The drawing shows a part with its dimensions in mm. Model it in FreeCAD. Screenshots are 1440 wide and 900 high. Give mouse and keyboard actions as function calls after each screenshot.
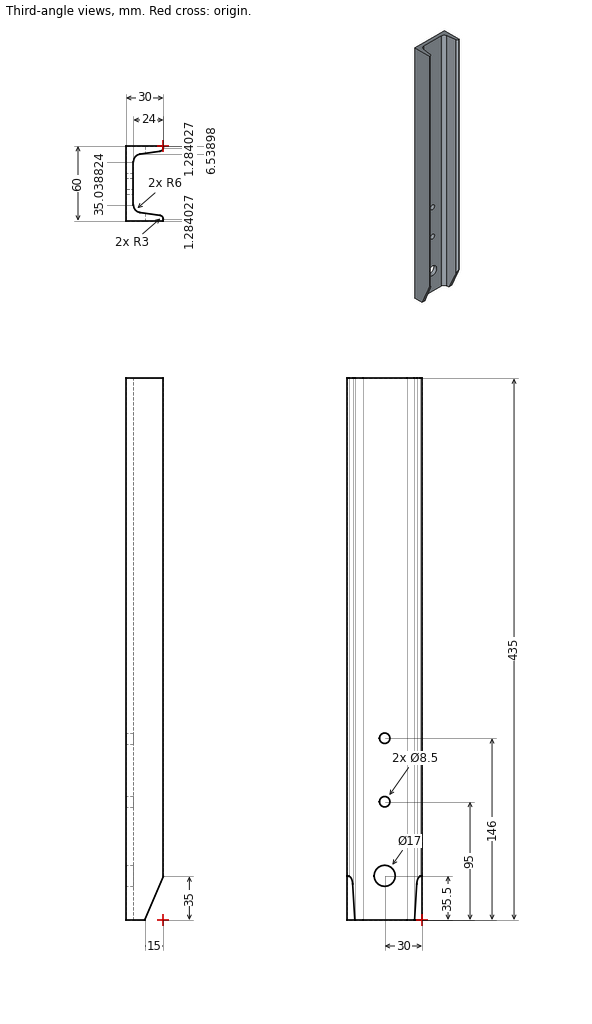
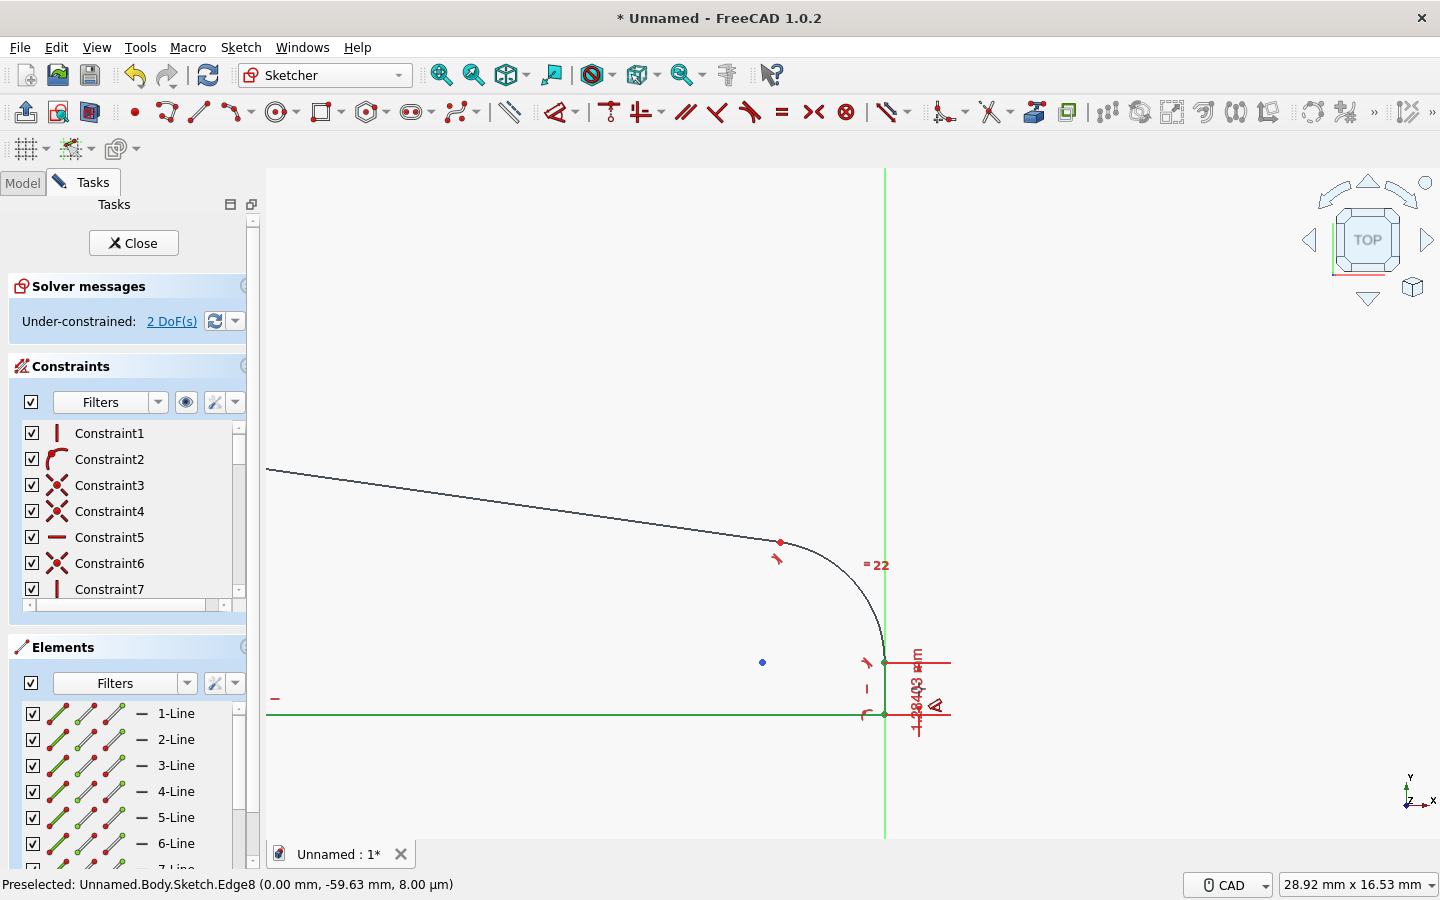
scroll(885, 703, down, 9)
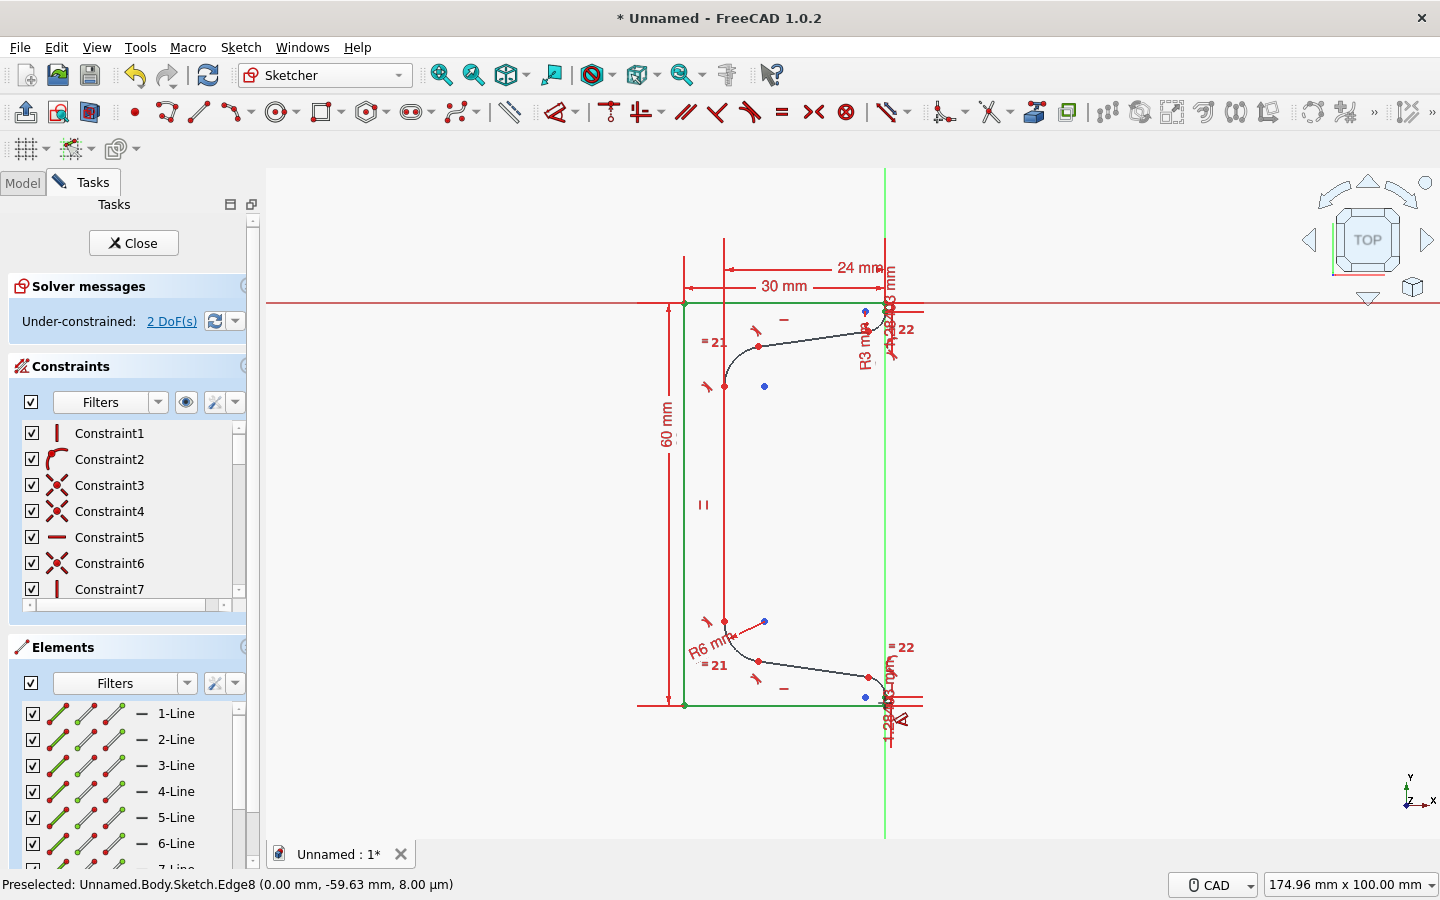
click(759, 347)
click(725, 325)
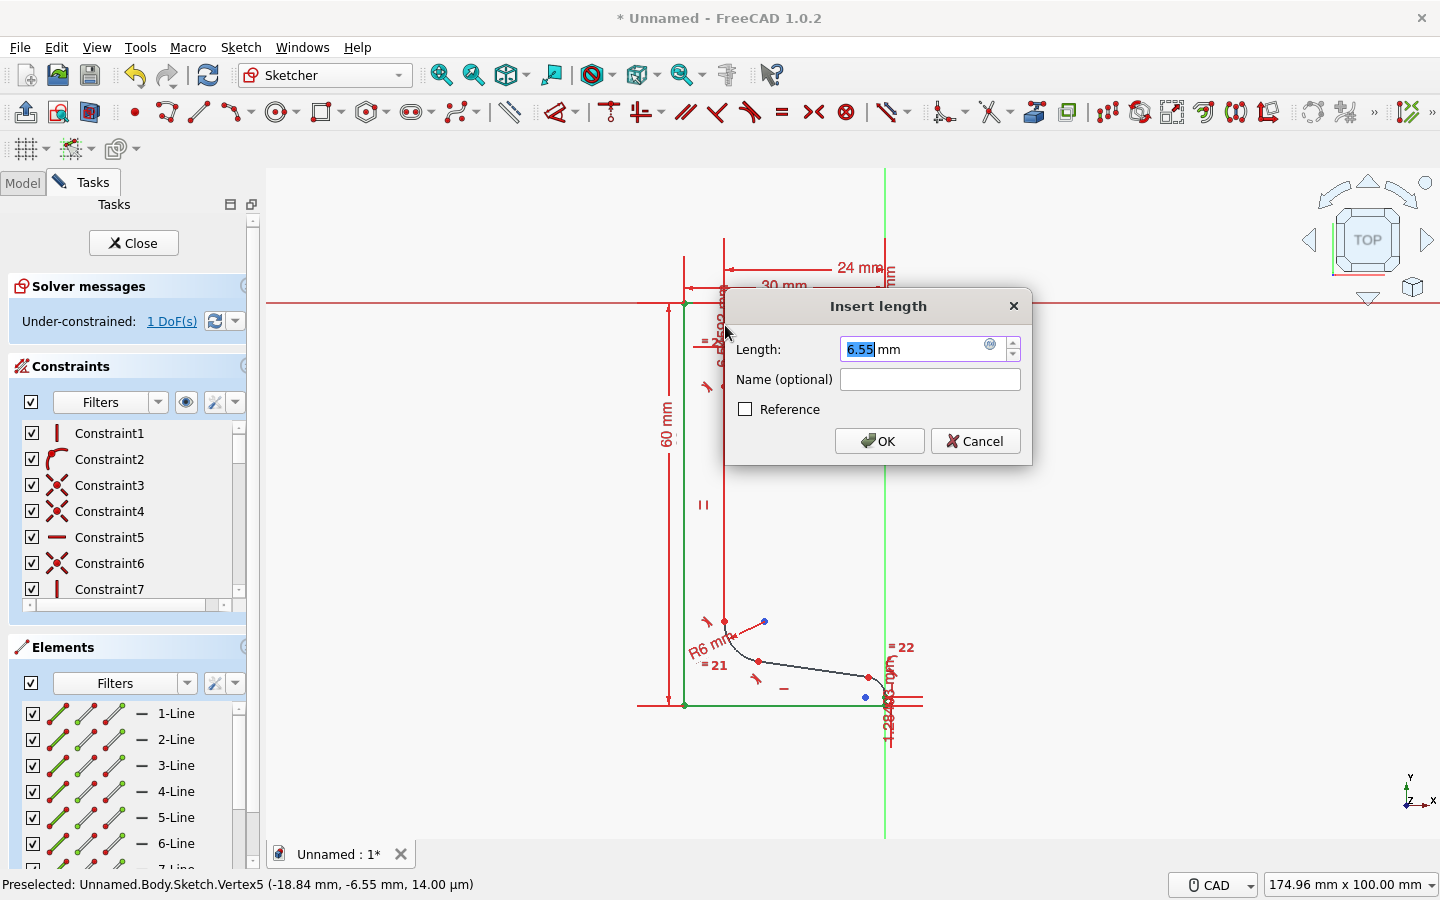
text(6.53898)
key(Return)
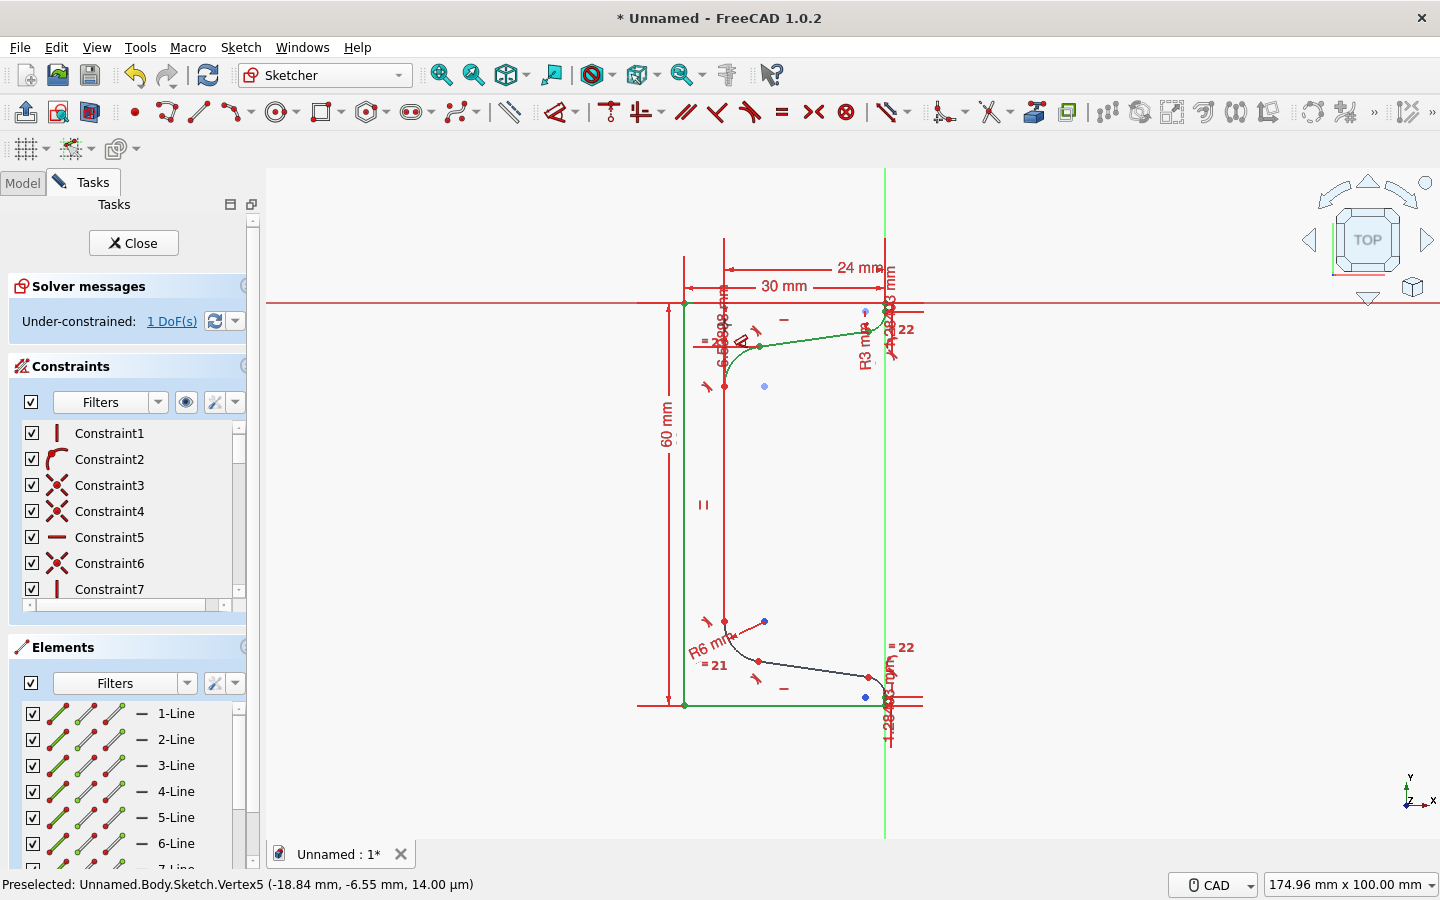
click(724, 551)
click(758, 504)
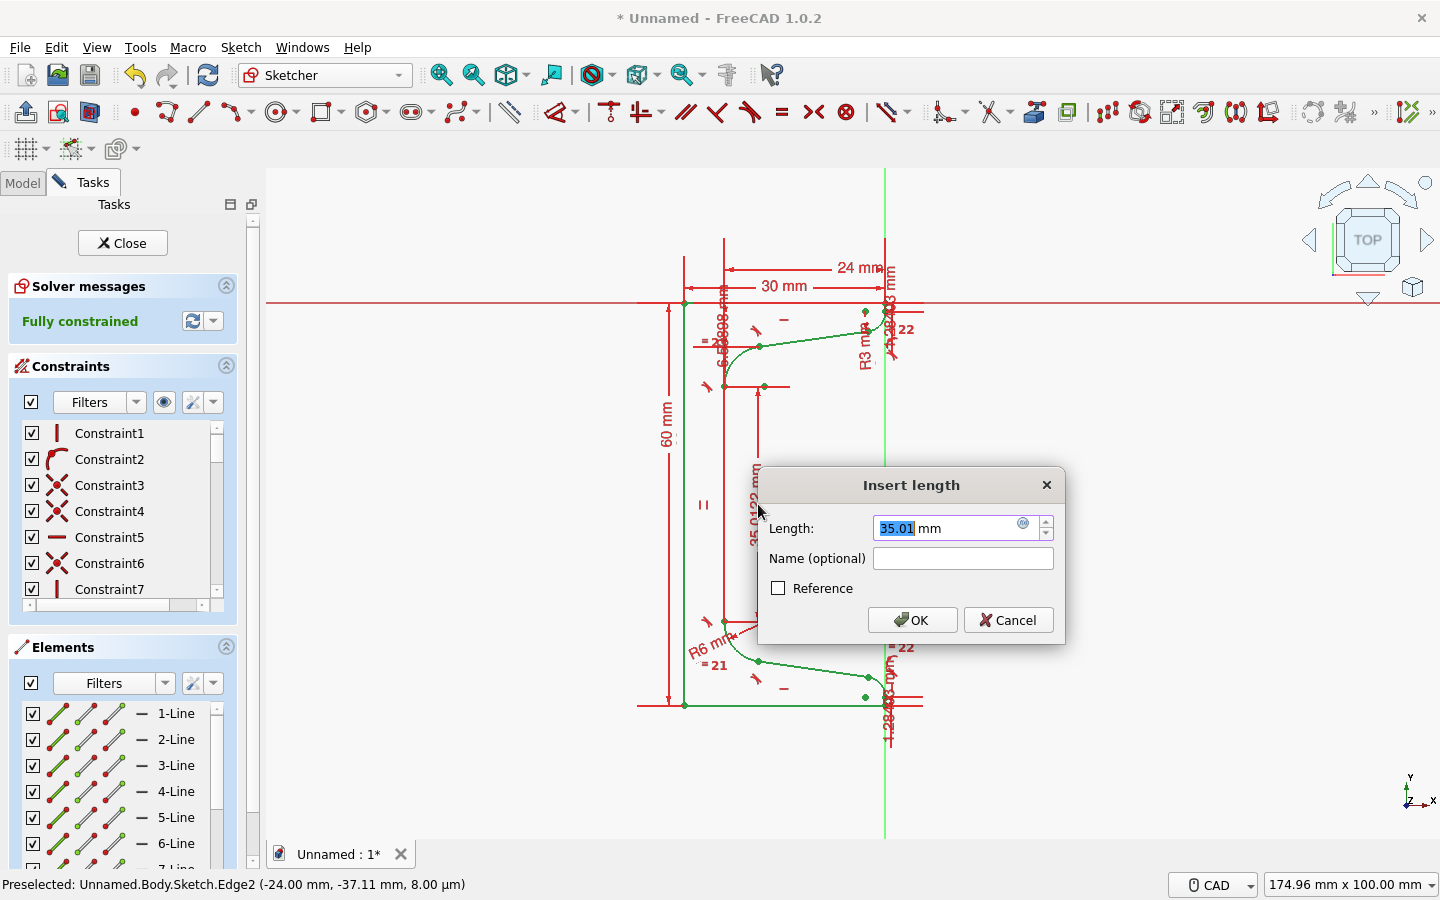
text(35.038824)
key(Return)
key(Escape)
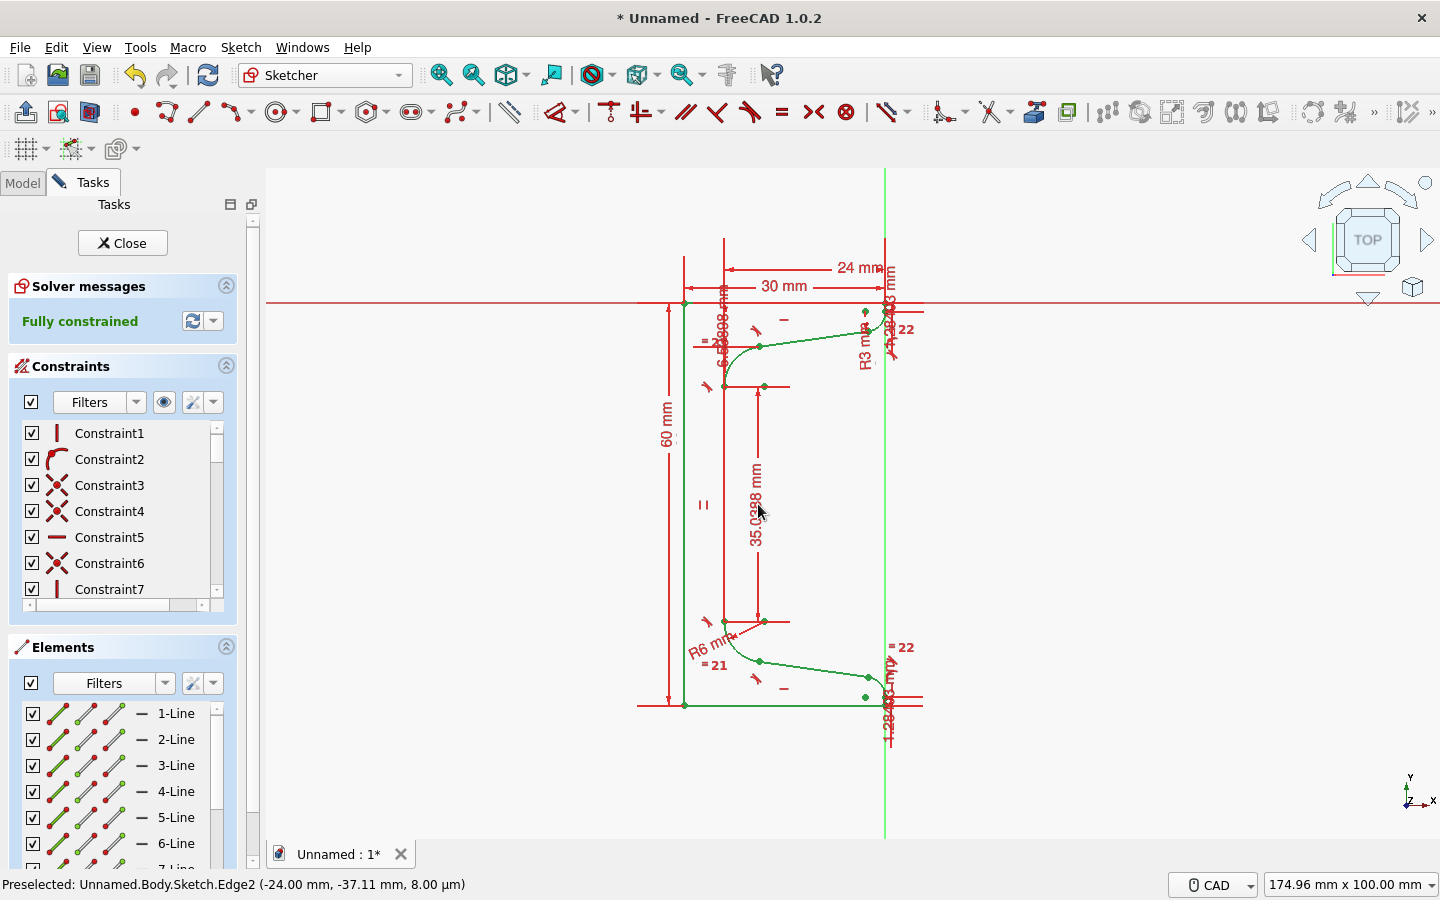
click(123, 243)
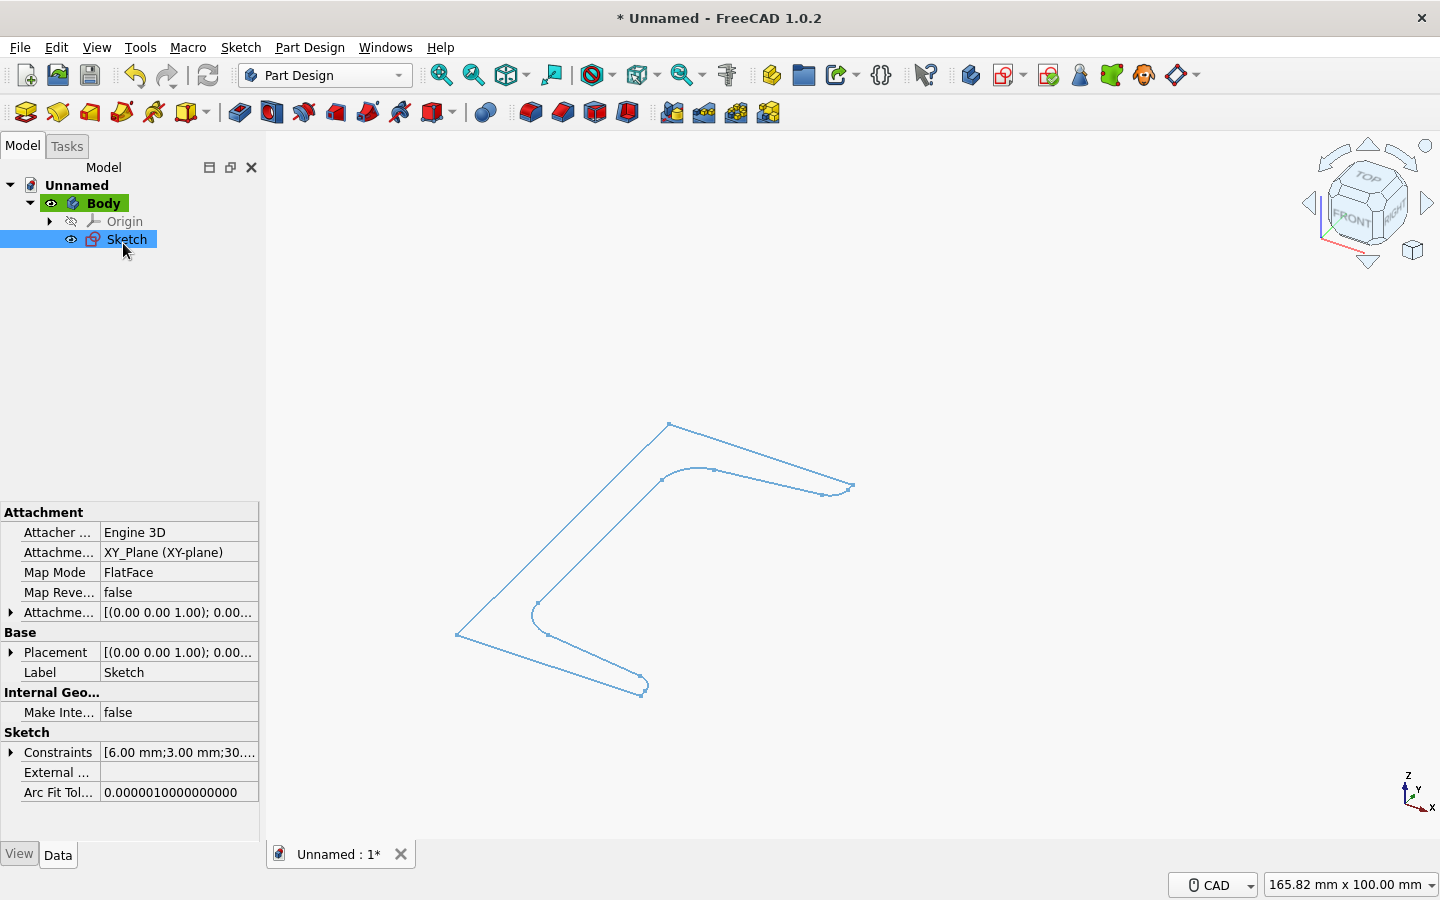
click(26, 112)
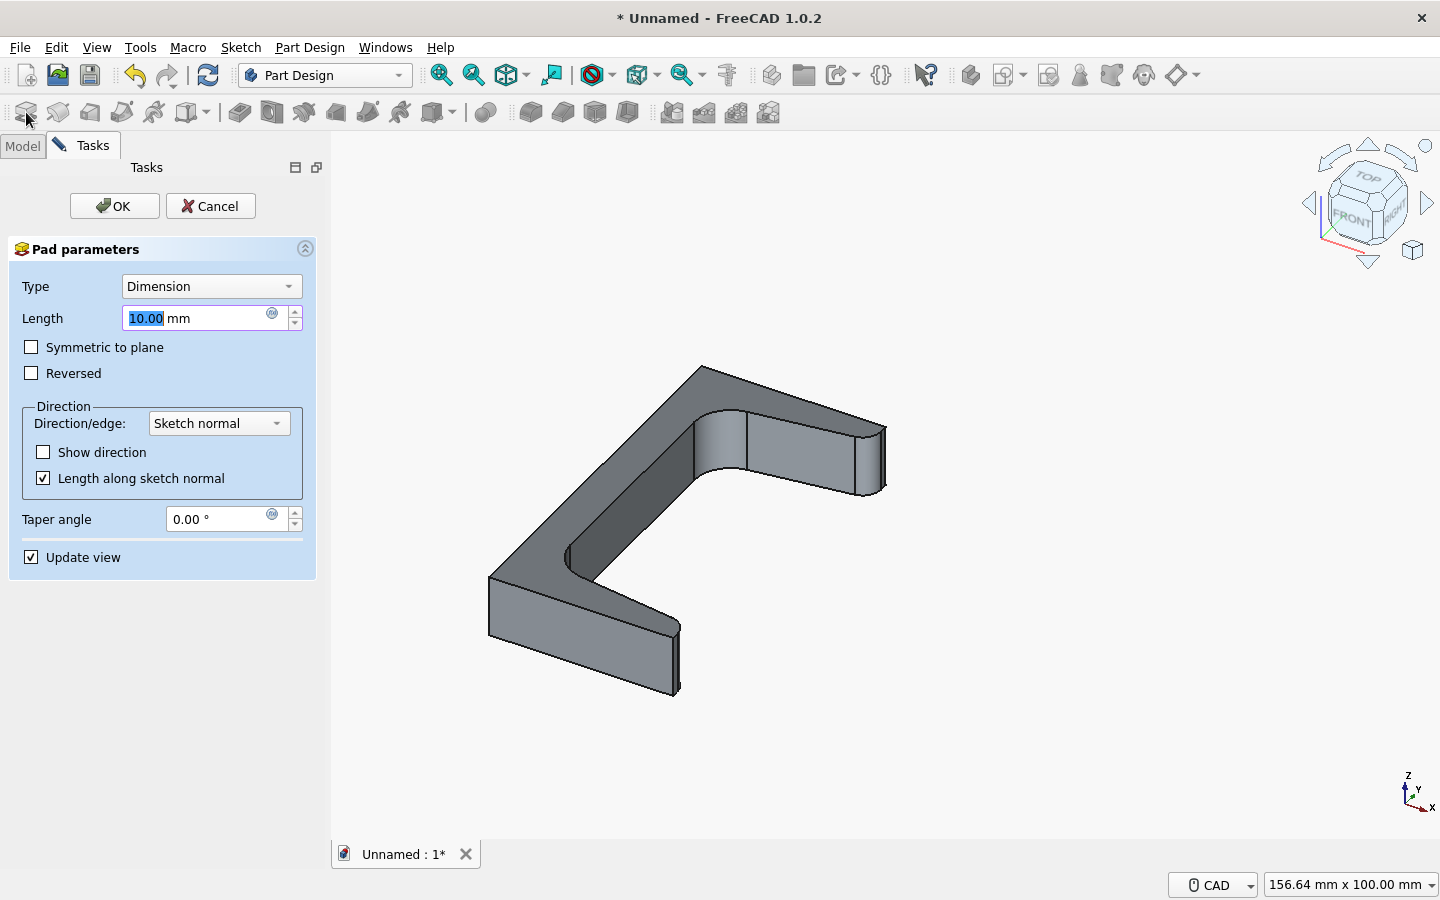
text(435)
key(Tab)